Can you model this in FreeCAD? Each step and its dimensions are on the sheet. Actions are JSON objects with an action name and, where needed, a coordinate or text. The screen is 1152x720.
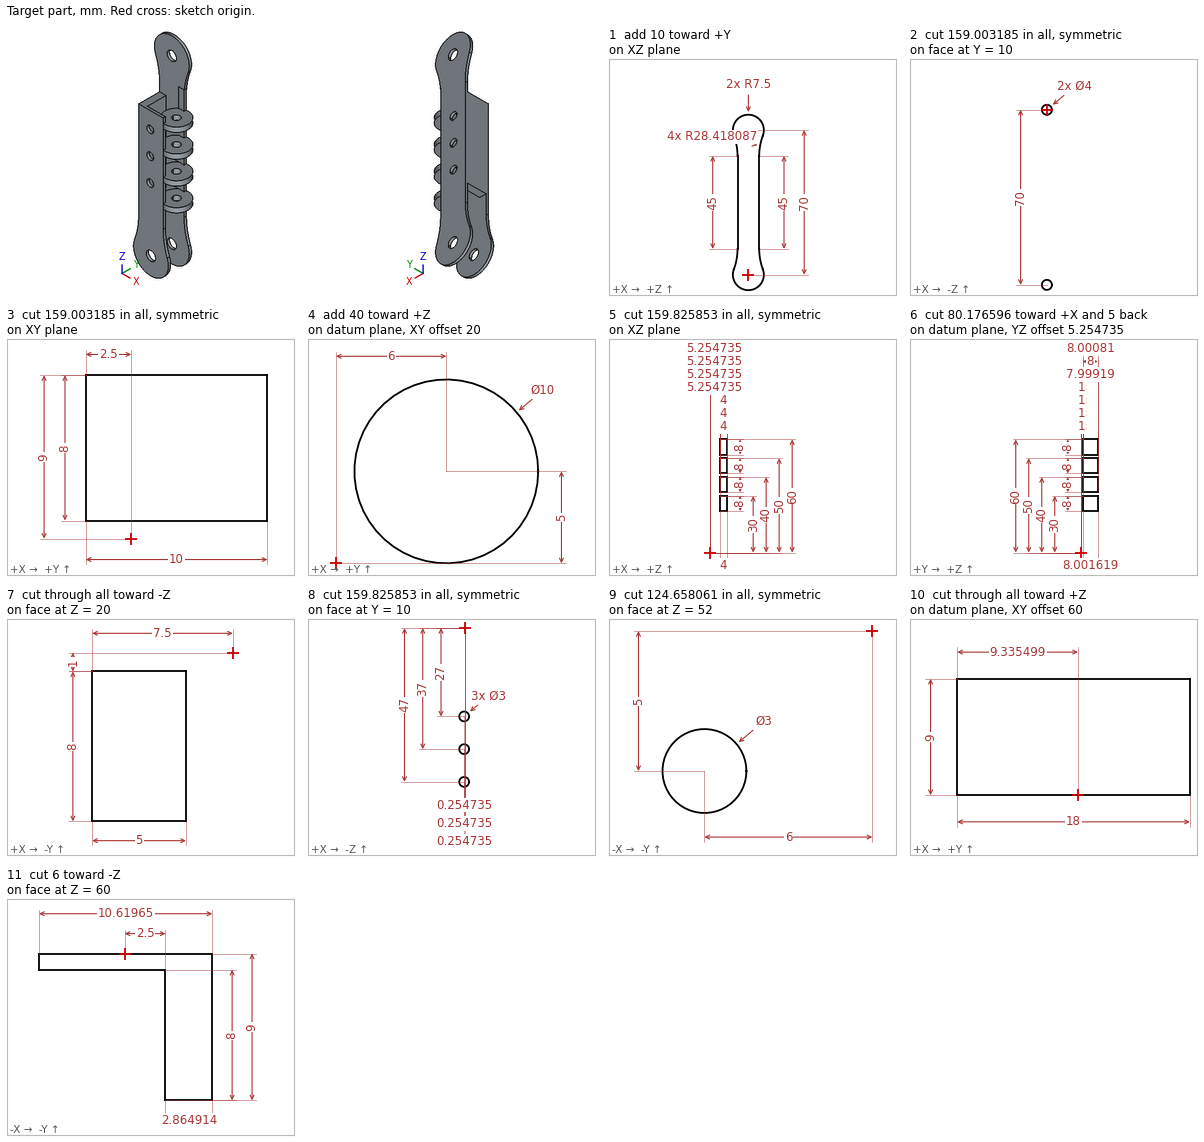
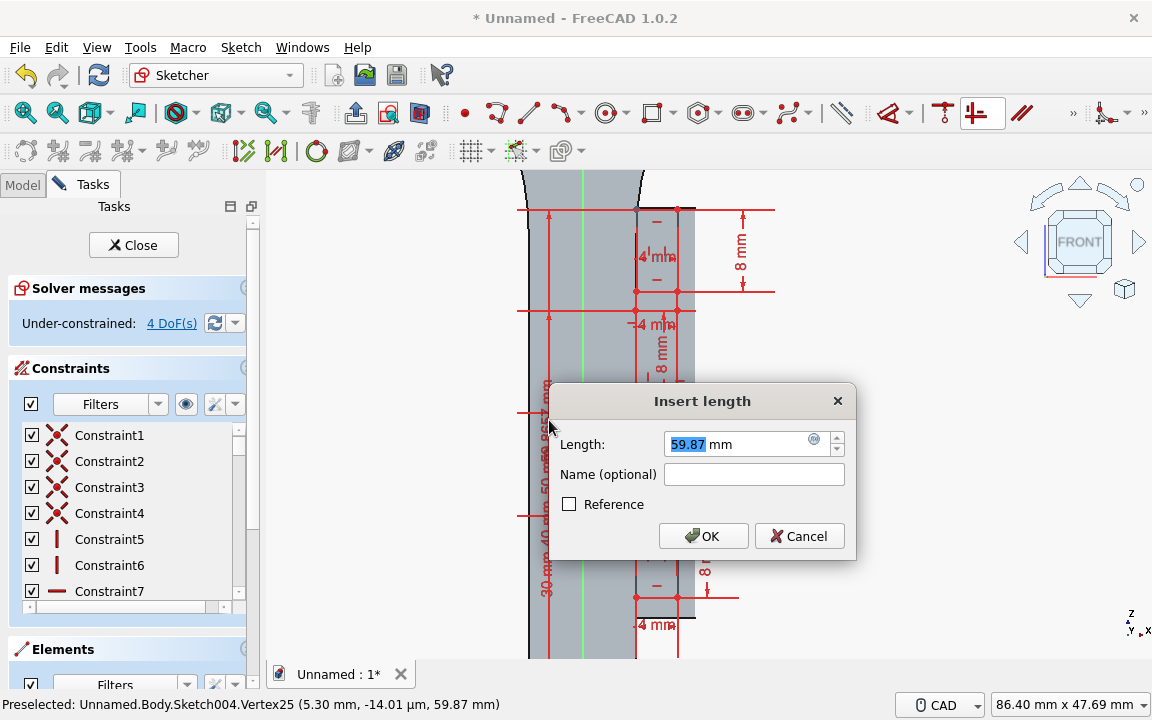
{"action": "type", "text": "60"}
{"action": "key", "text": "Return"}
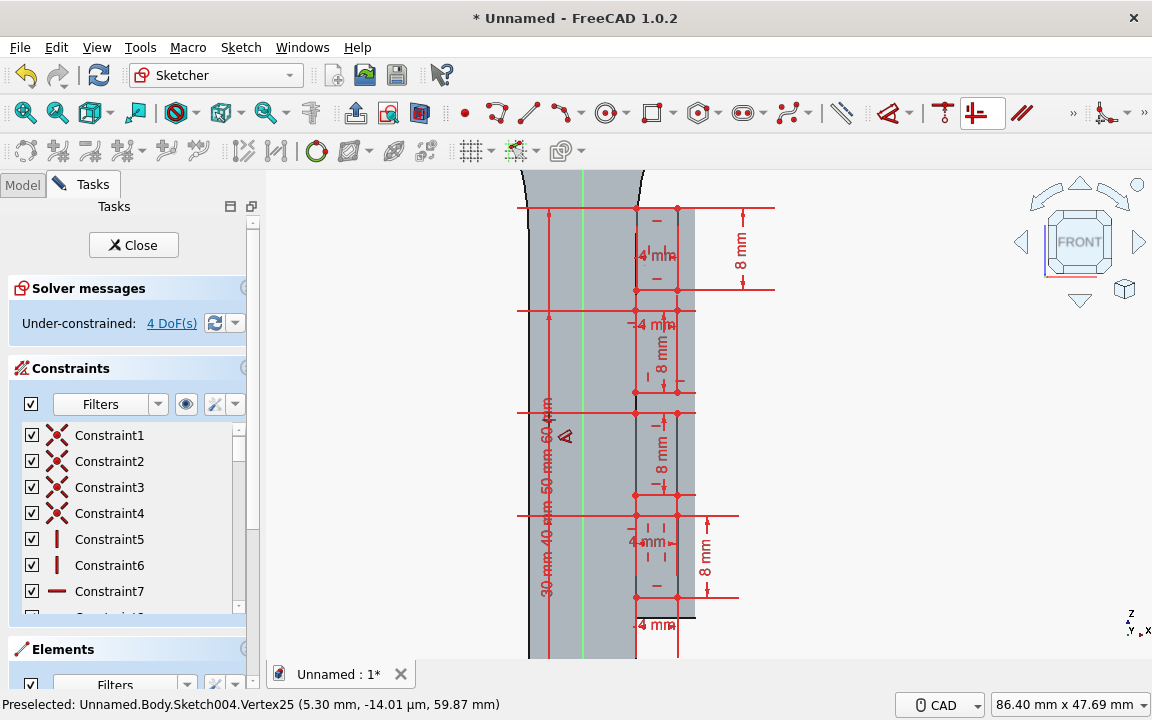
{"action": "left_click", "coordinate": [636, 516]}
{"action": "left_click", "coordinate": [622, 482]}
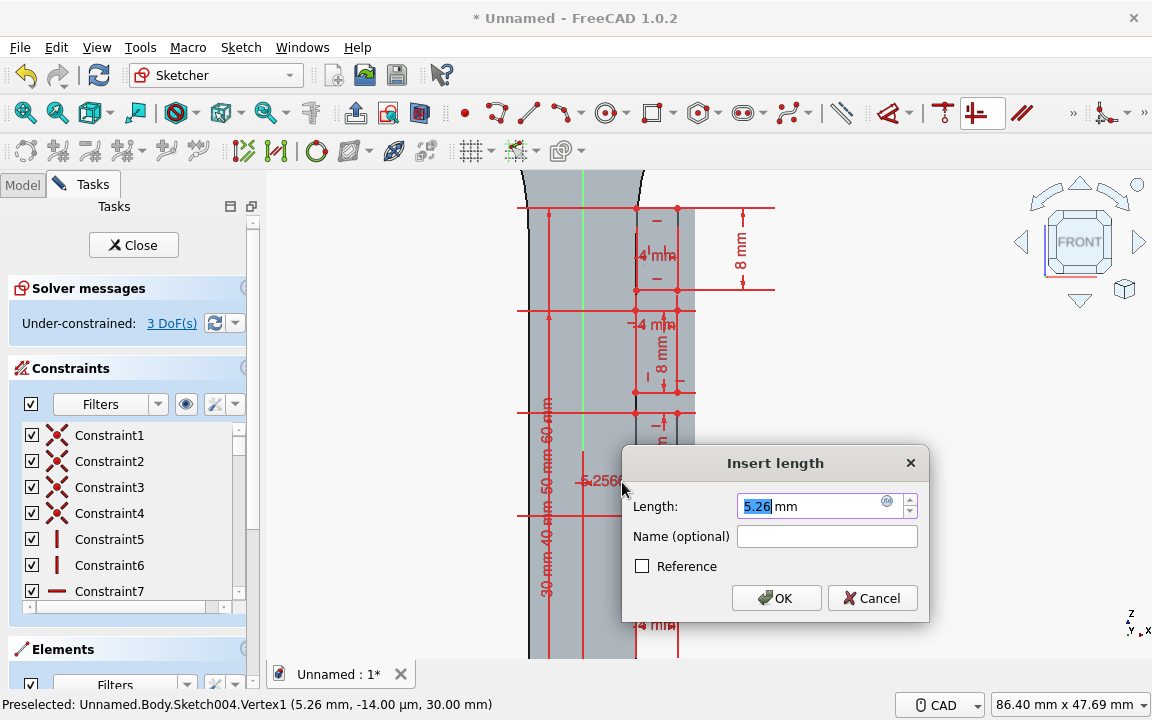
{"action": "type", "text": "5.254735"}
{"action": "key", "text": "Return"}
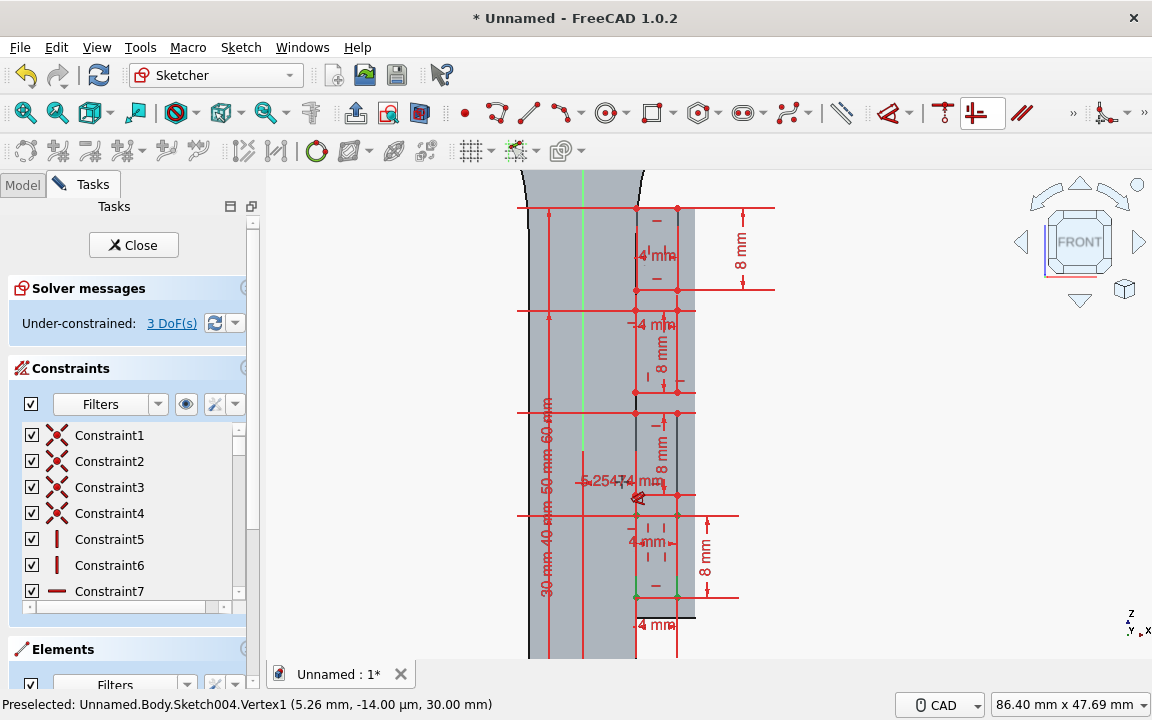
{"action": "left_click", "coordinate": [636, 413]}
{"action": "left_click", "coordinate": [609, 379]}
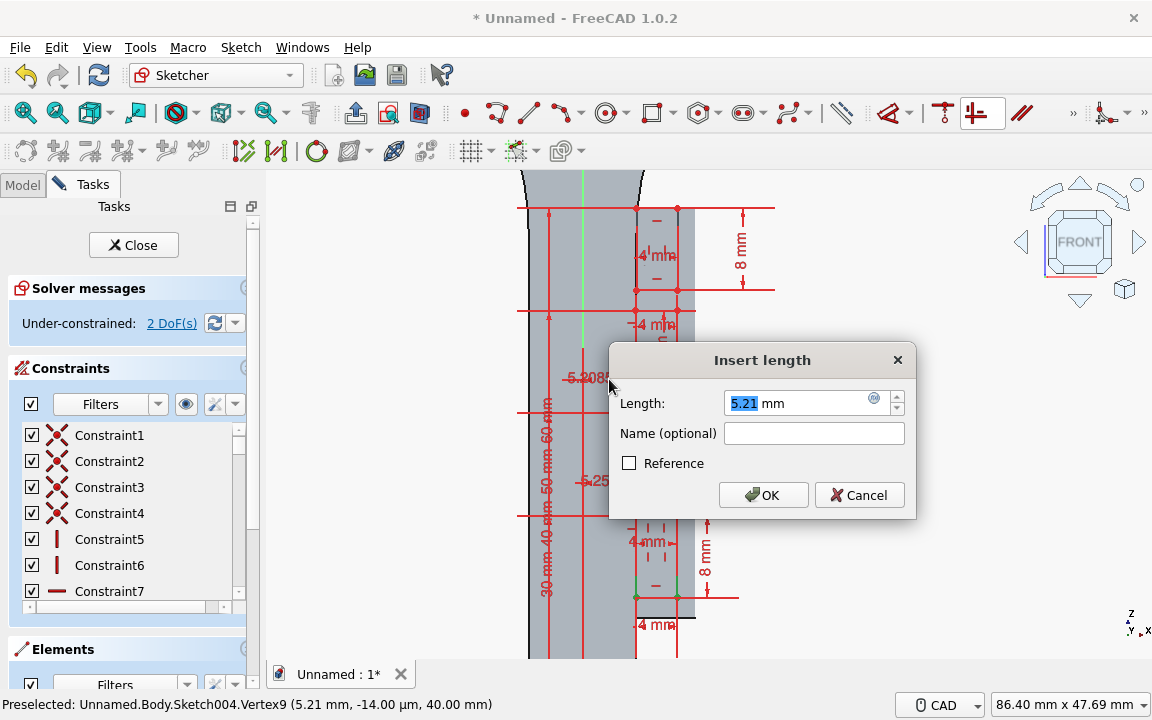
{"action": "type", "text": "5.254735"}
{"action": "key", "text": "Return"}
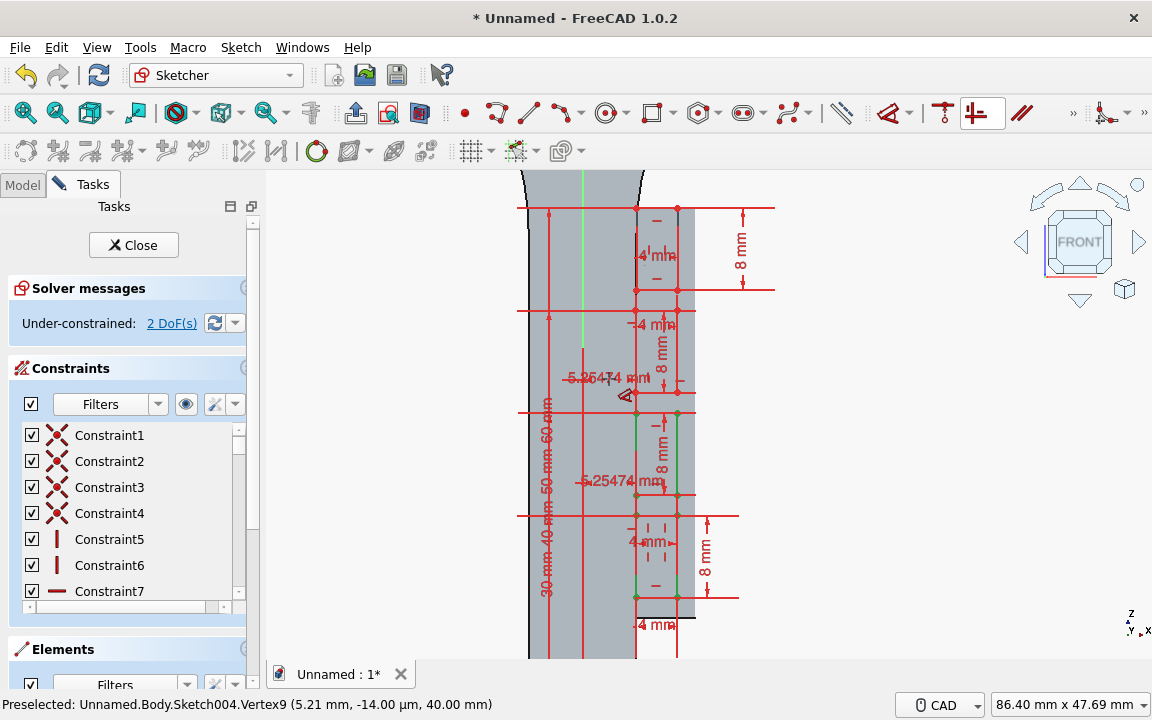
{"action": "left_click", "coordinate": [636, 311]}
{"action": "left_click", "coordinate": [609, 229]}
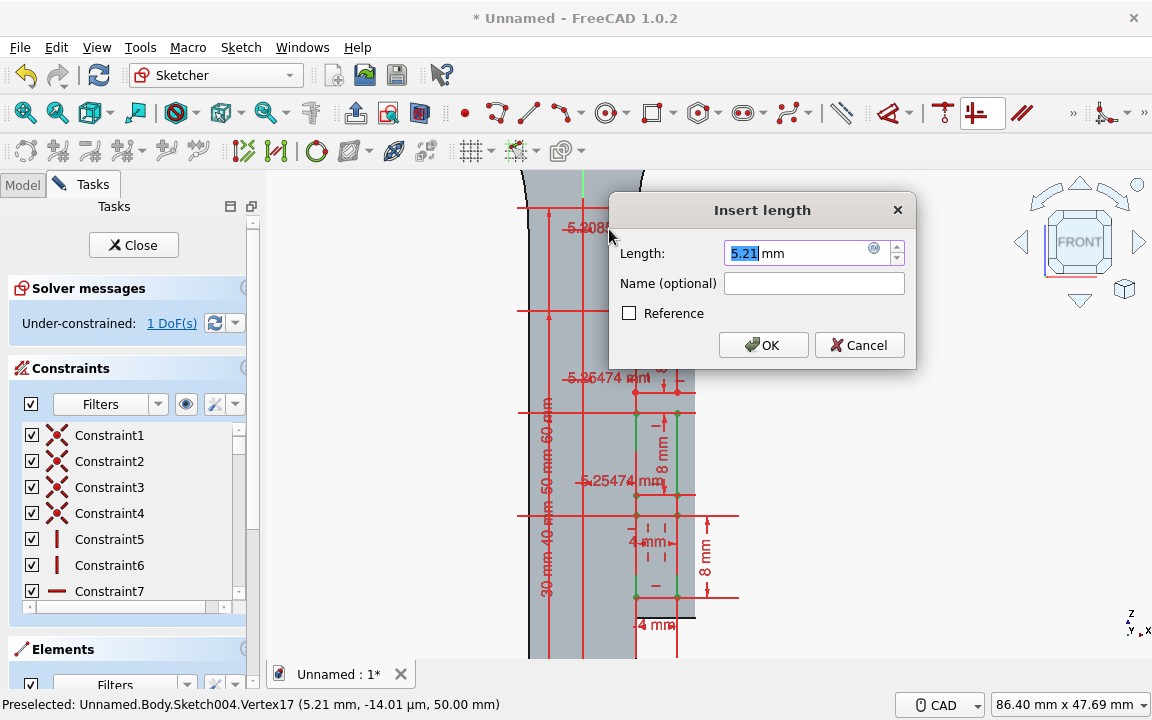
{"action": "type", "text": "5.254735"}
{"action": "key", "text": "Return"}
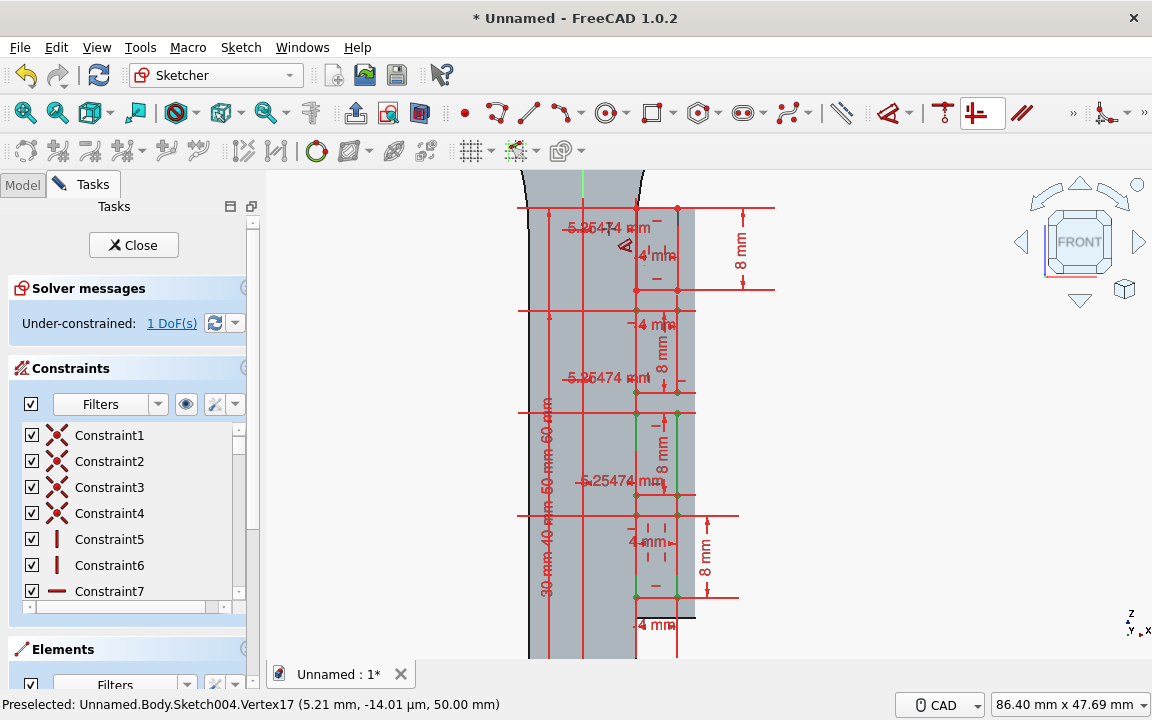
{"action": "left_click", "coordinate": [637, 208]}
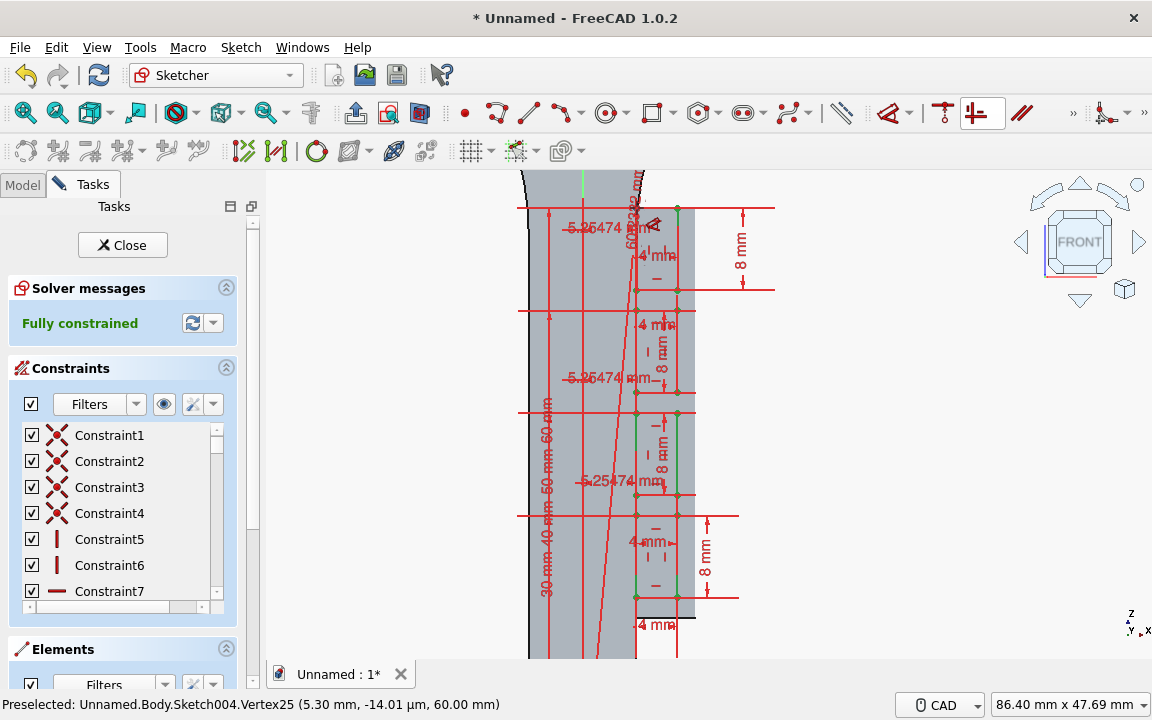
{"action": "key", "text": "Escape"}
{"action": "key", "text": "Escape"}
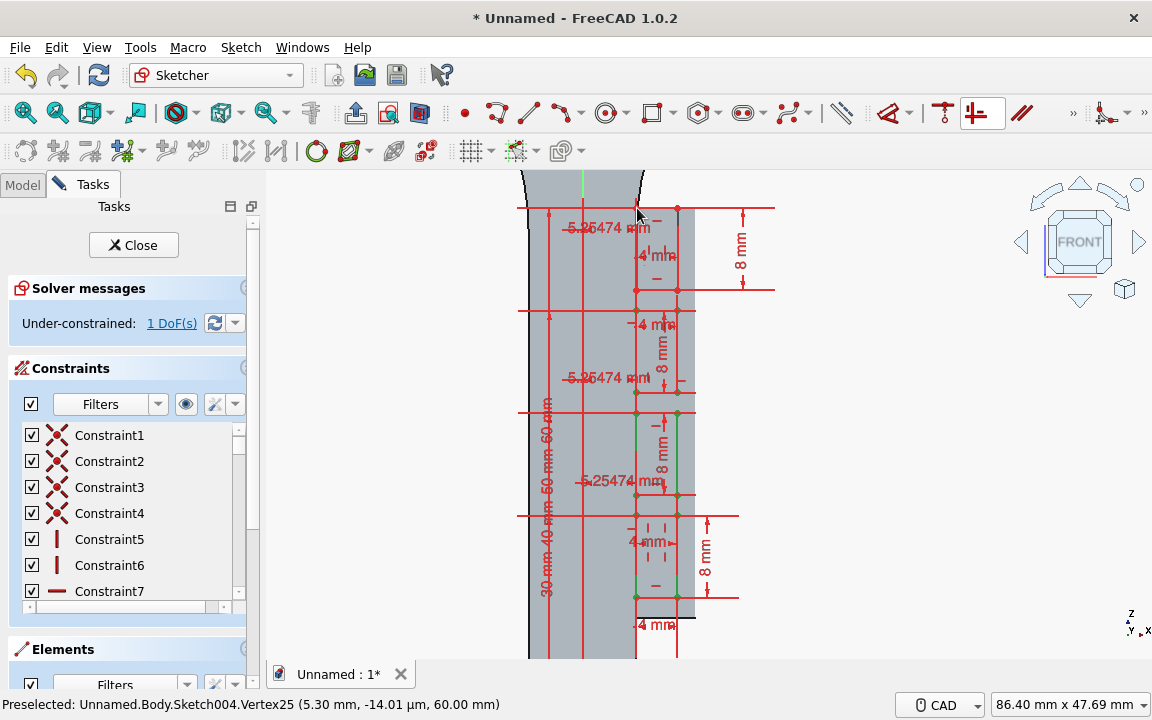
{"action": "left_click", "coordinate": [637, 208]}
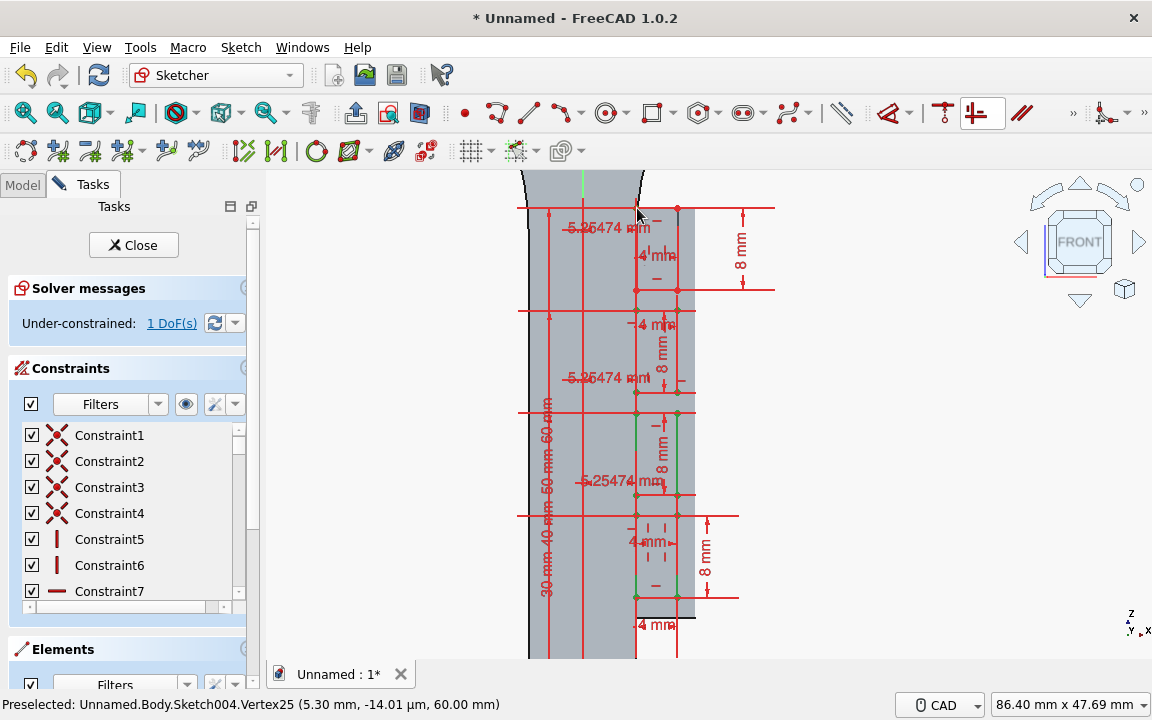
{"action": "key", "text": "l"}